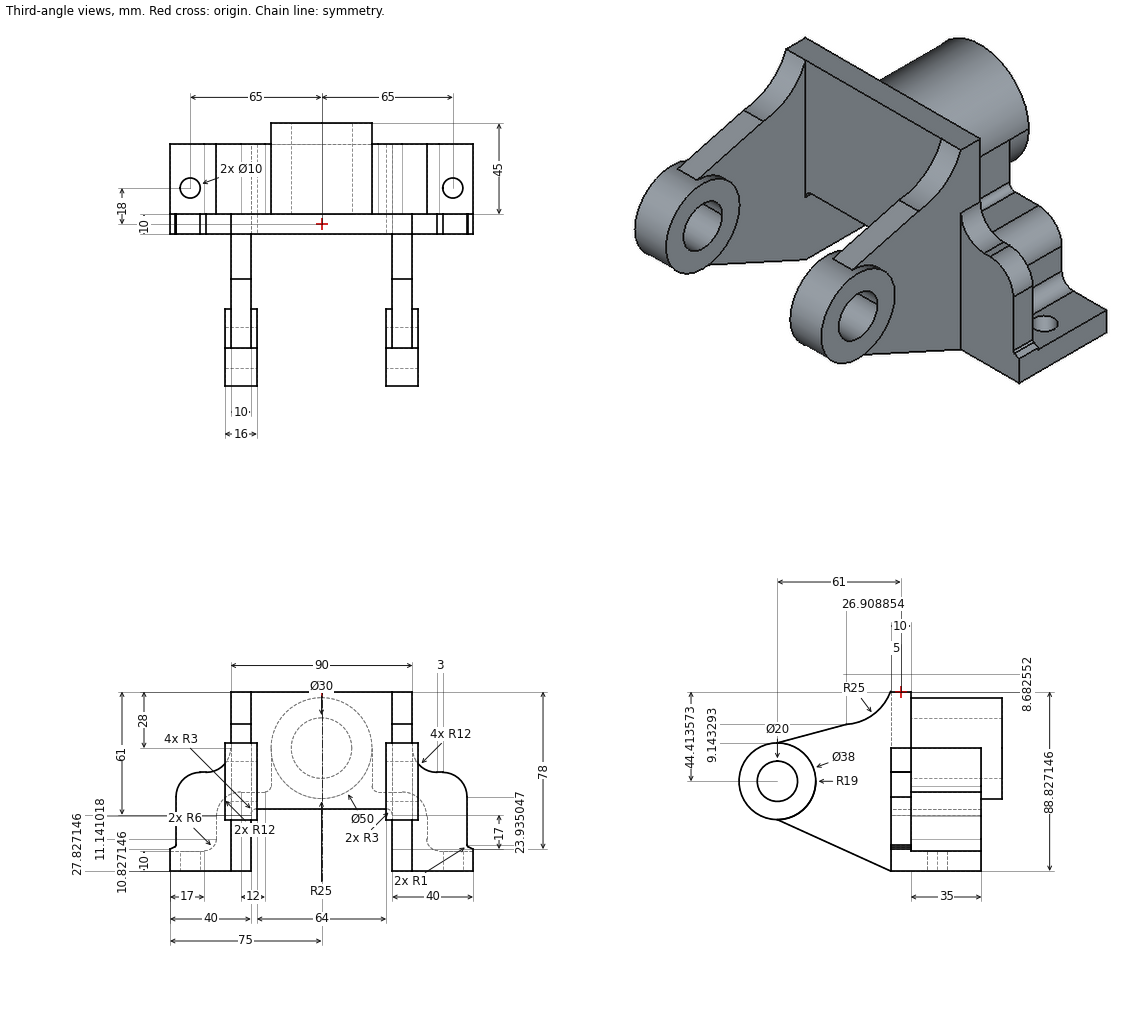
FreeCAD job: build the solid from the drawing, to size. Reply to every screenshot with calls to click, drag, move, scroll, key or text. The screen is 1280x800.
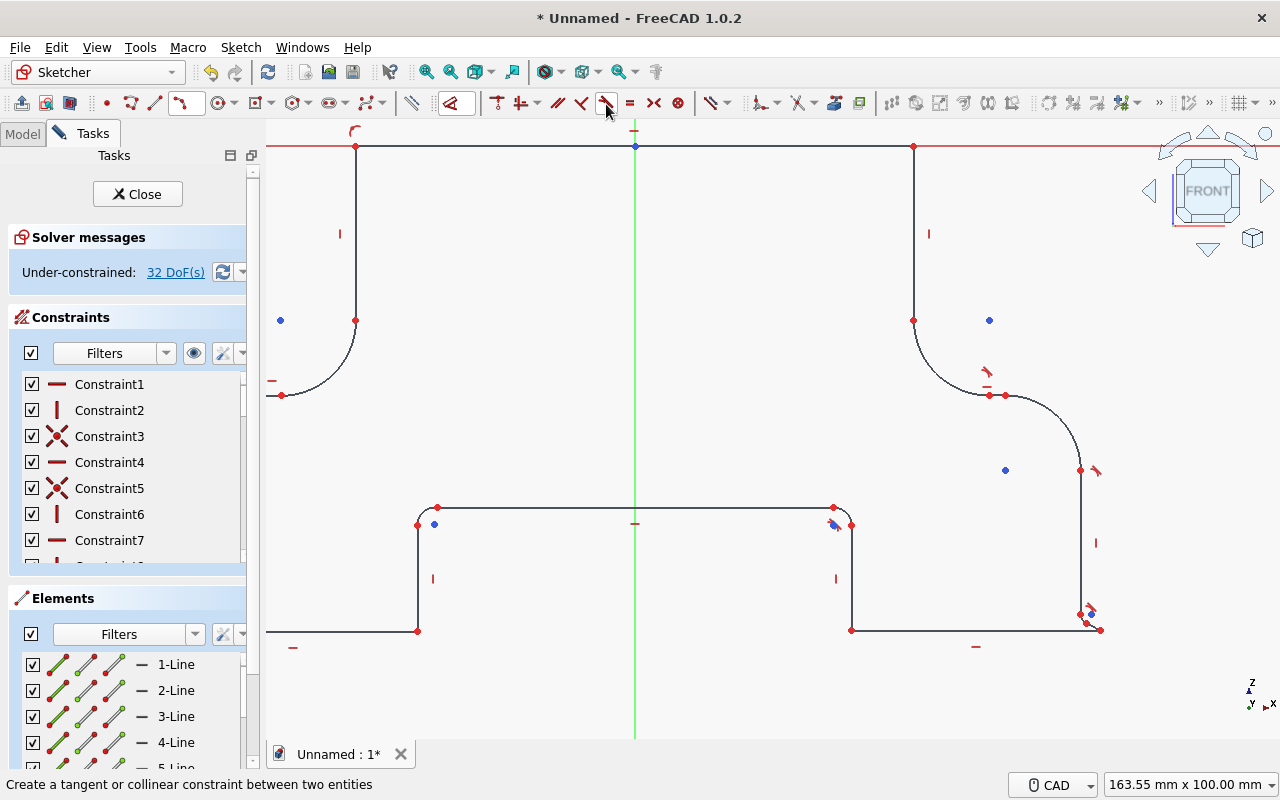
click(715, 508)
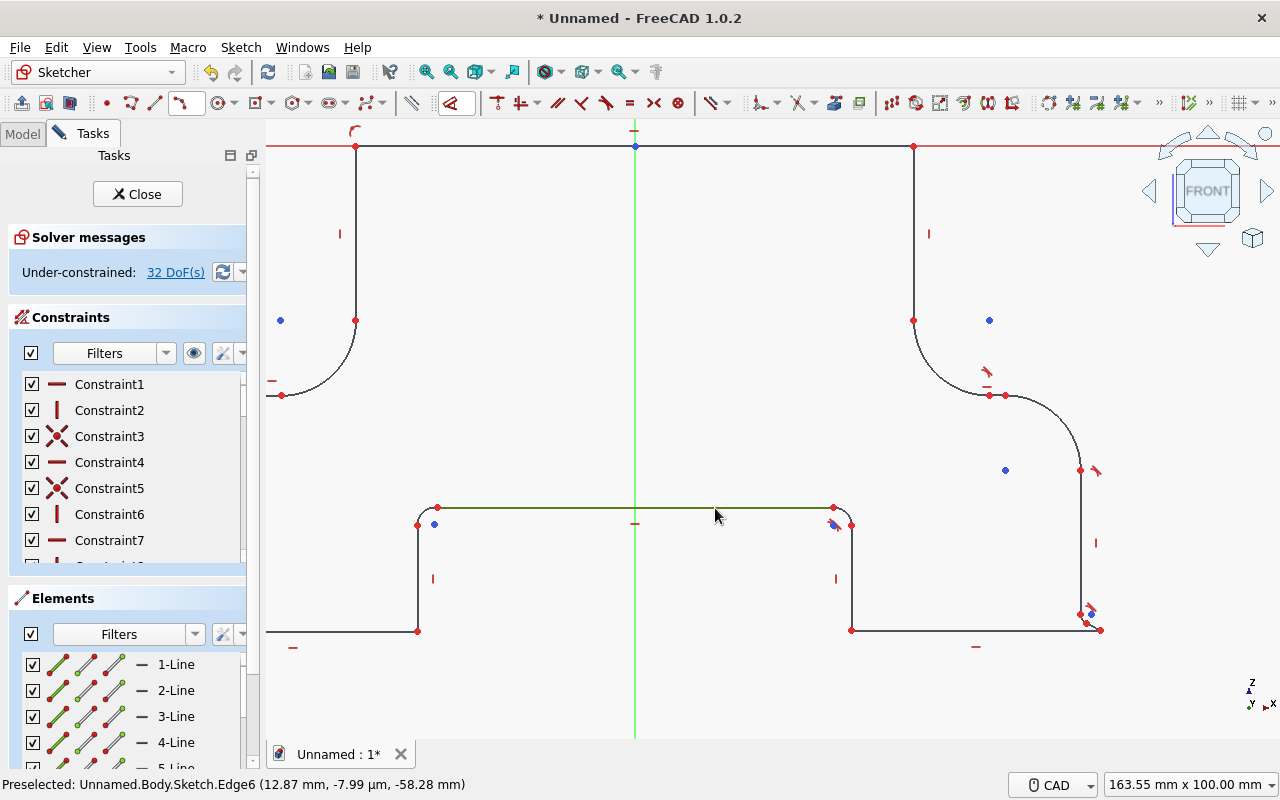
click(423, 512)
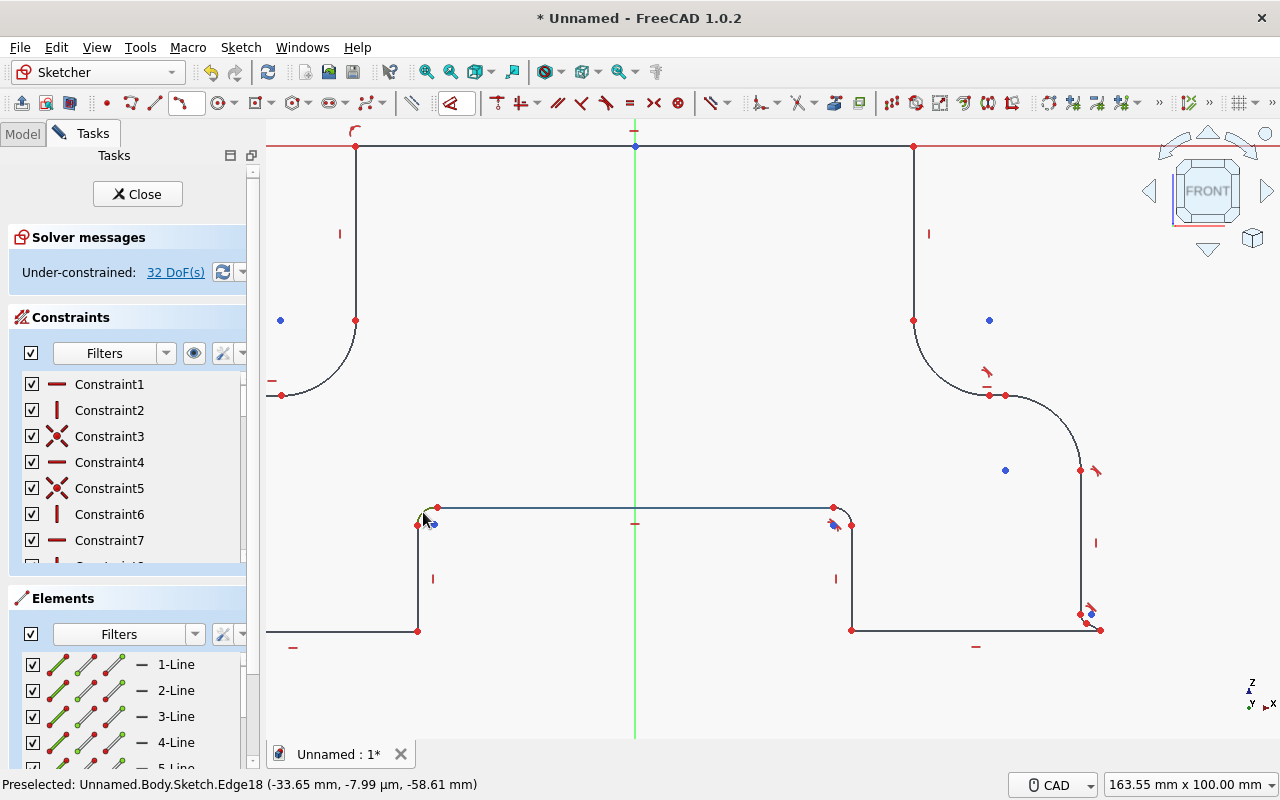
key(t)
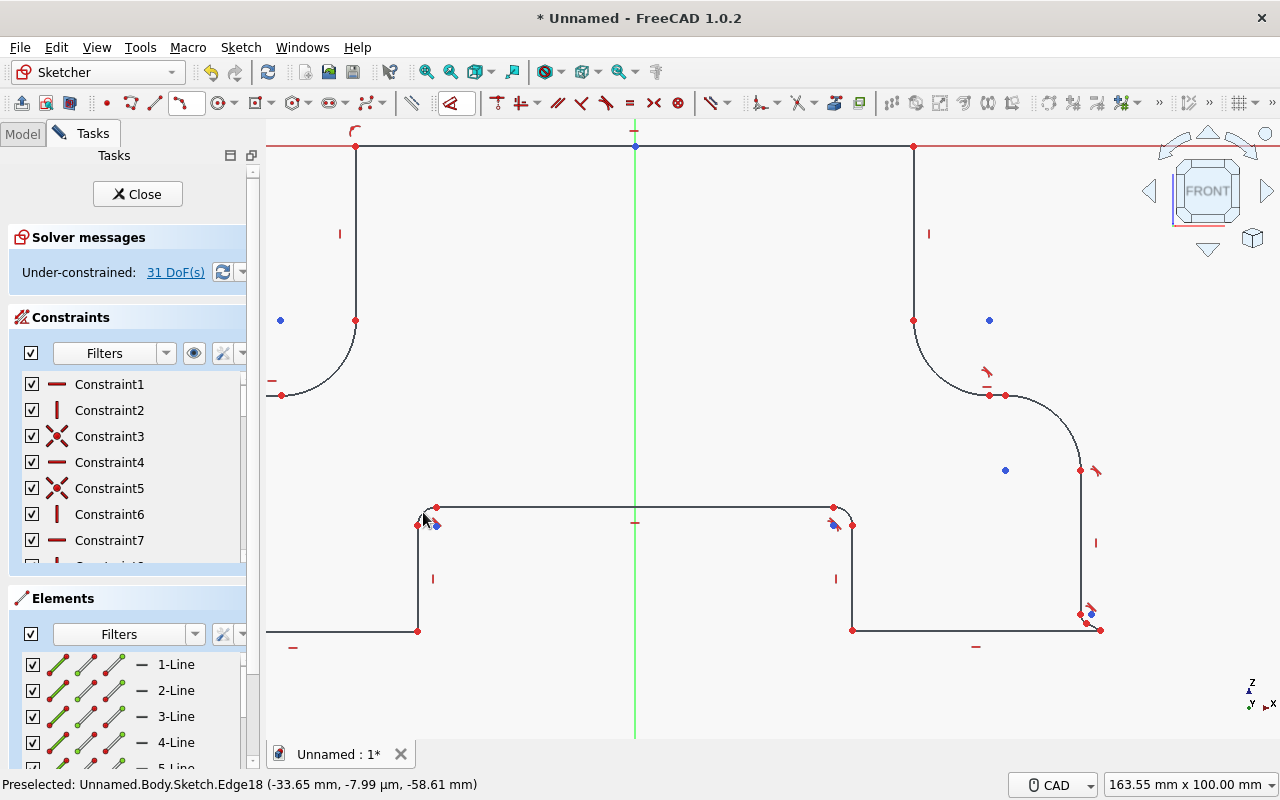
click(418, 557)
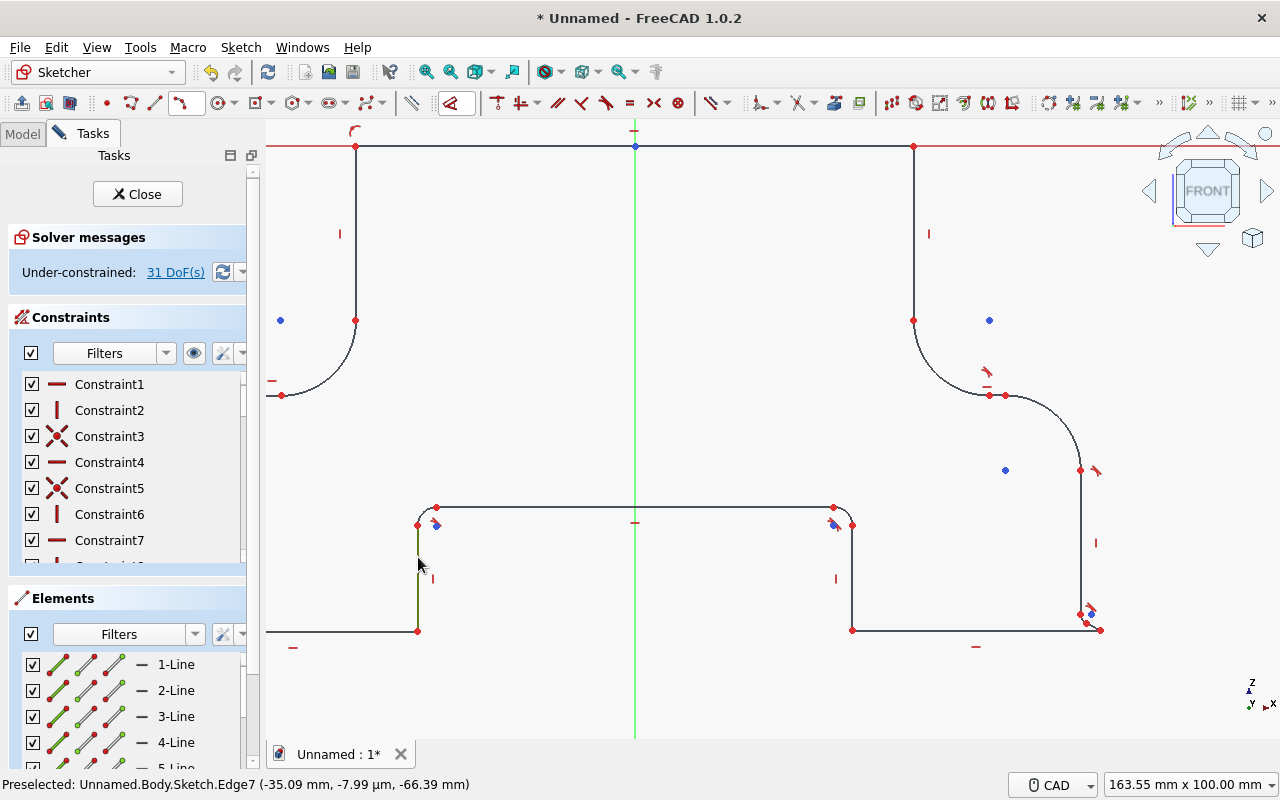
click(424, 512)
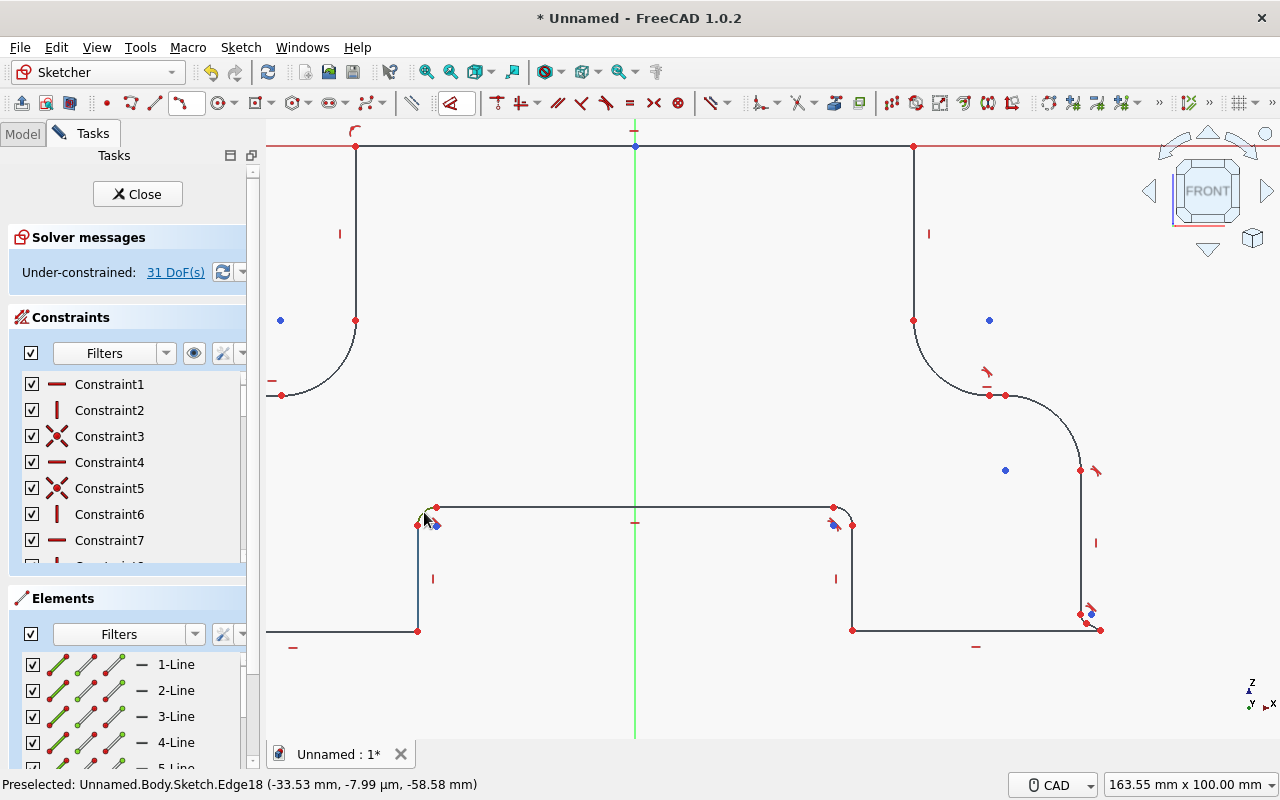
click(606, 104)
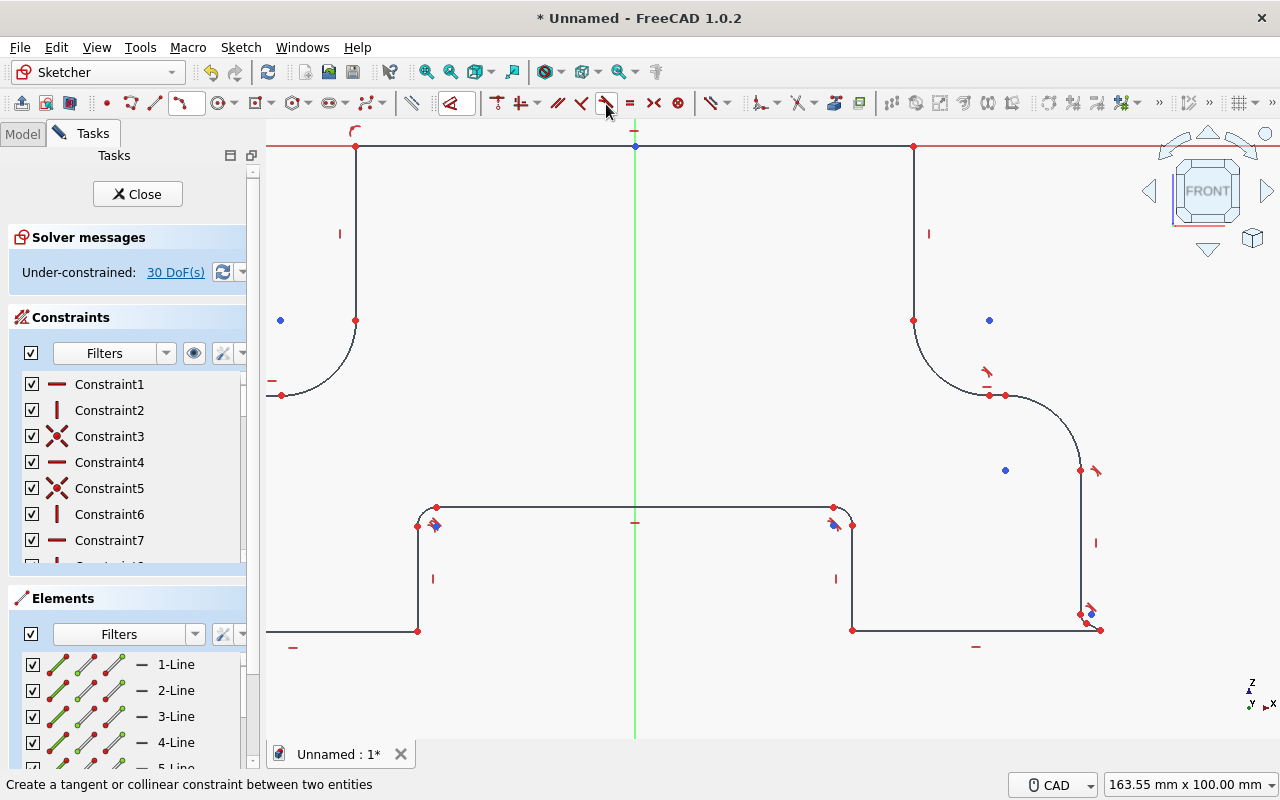
scroll(845, 512, down, 2)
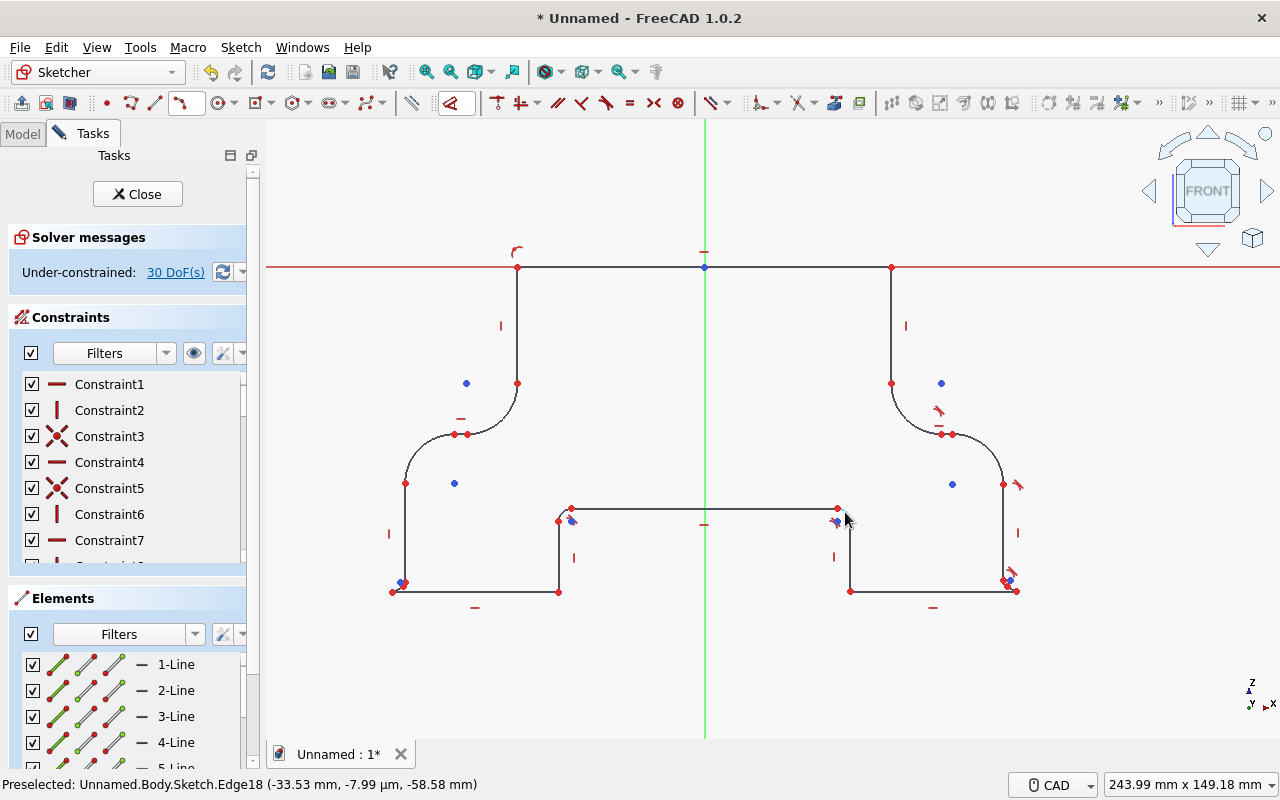
scroll(400, 589, up, 7)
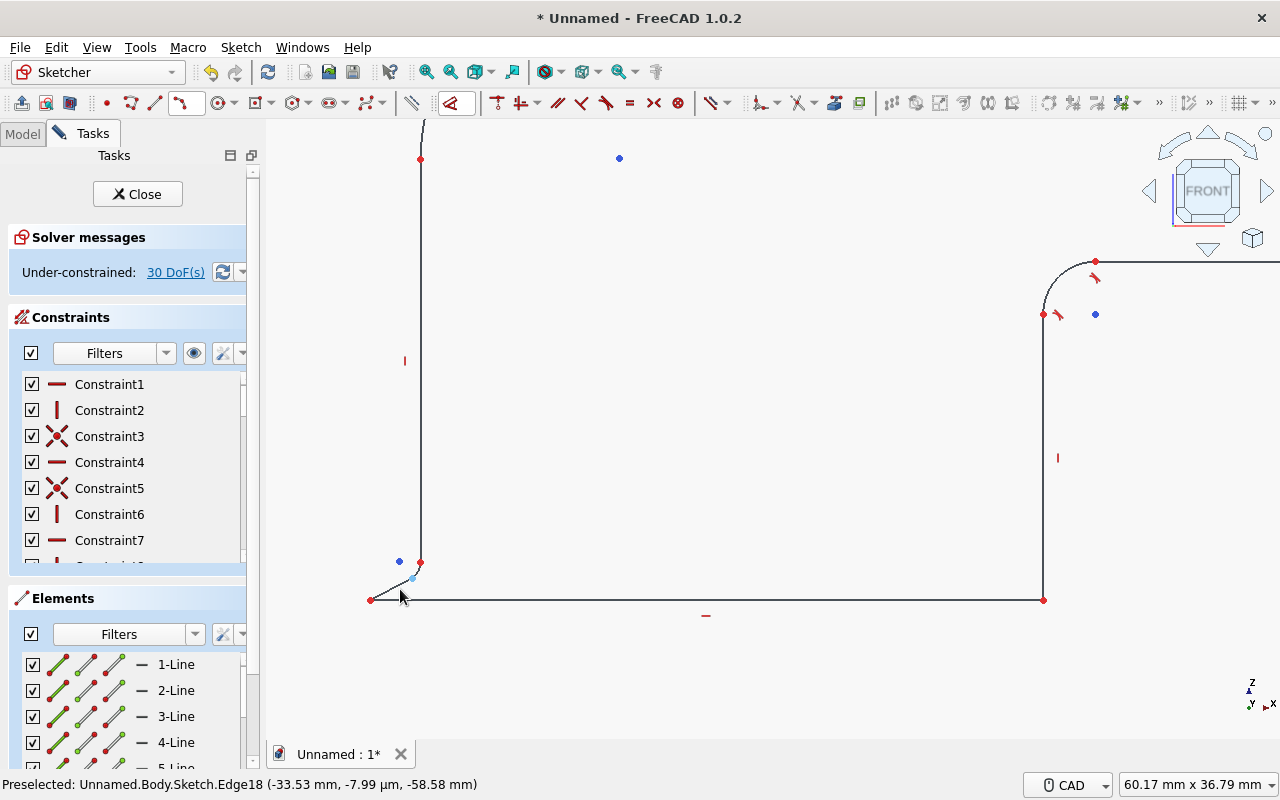
click(400, 585)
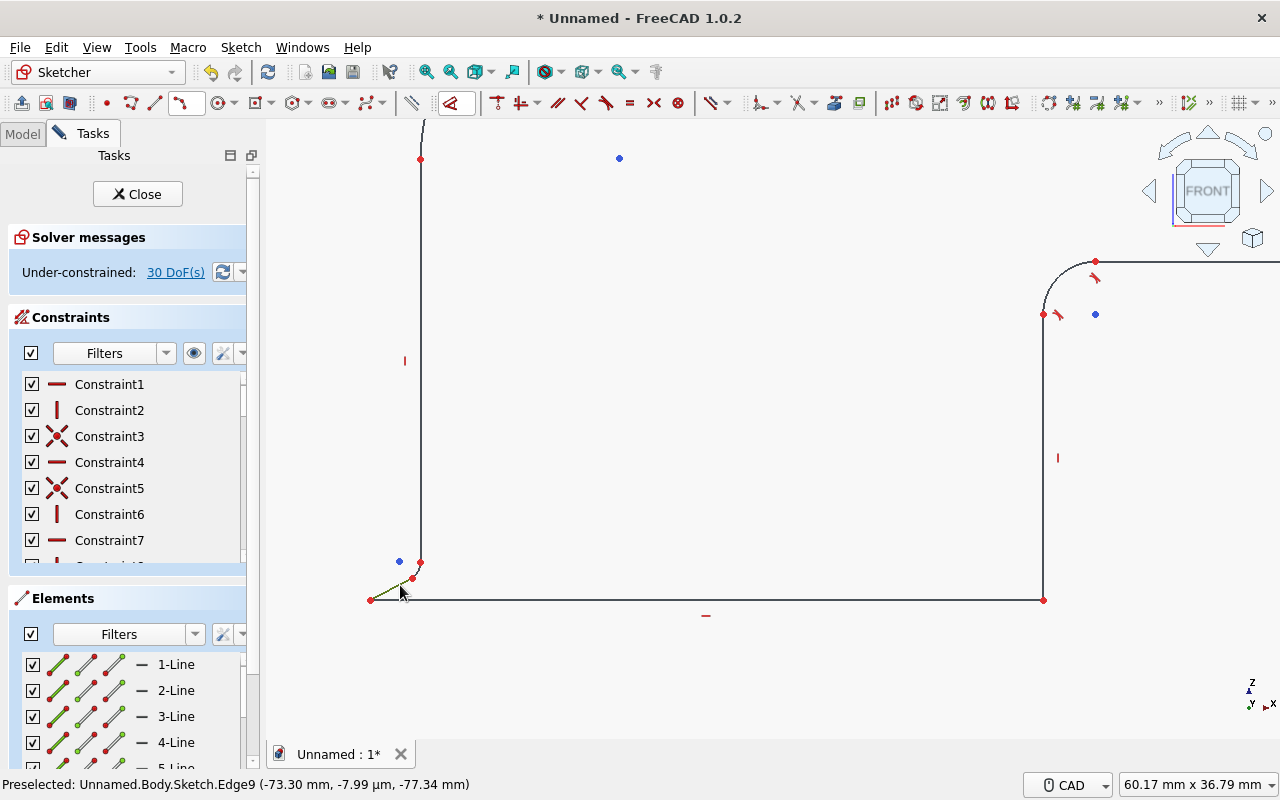
scroll(418, 571, up, 3)